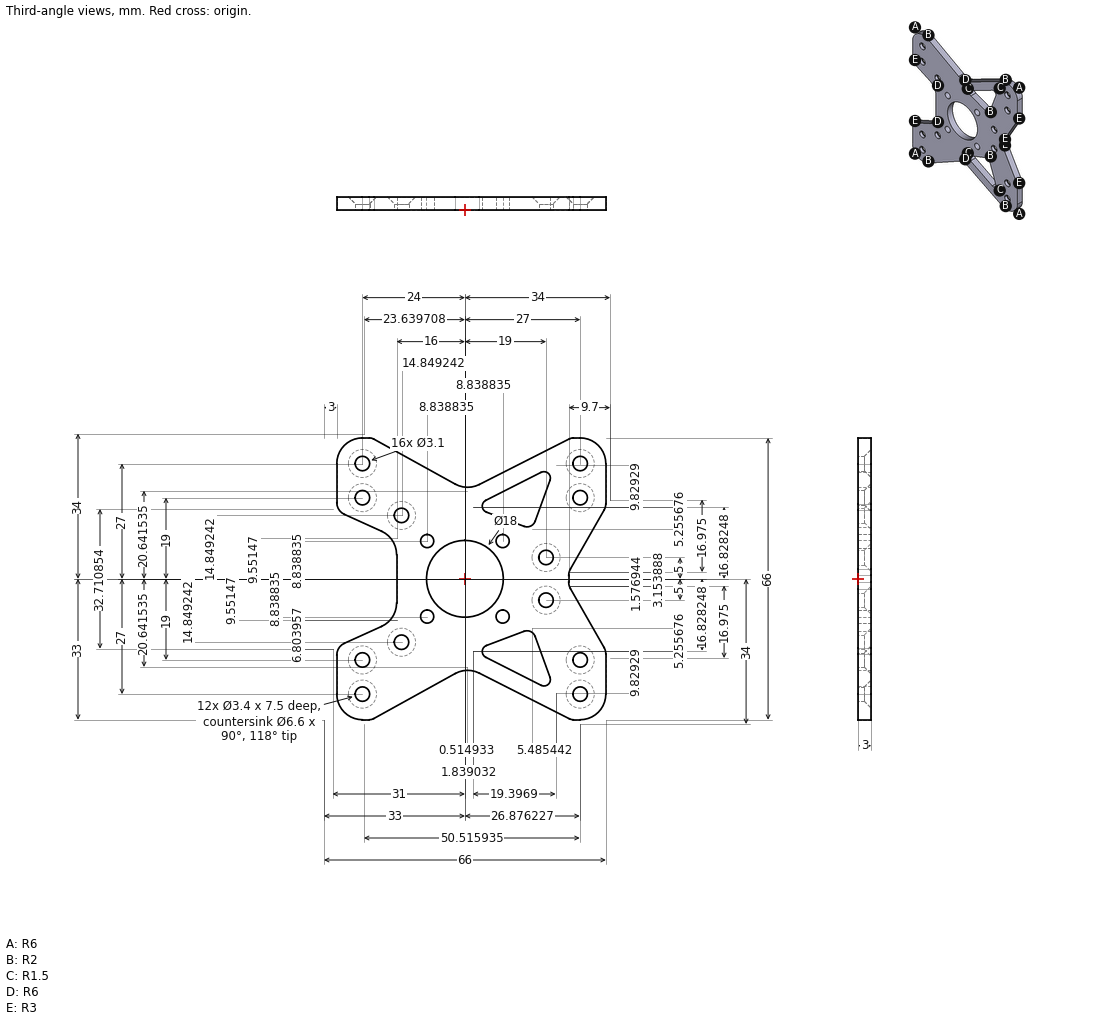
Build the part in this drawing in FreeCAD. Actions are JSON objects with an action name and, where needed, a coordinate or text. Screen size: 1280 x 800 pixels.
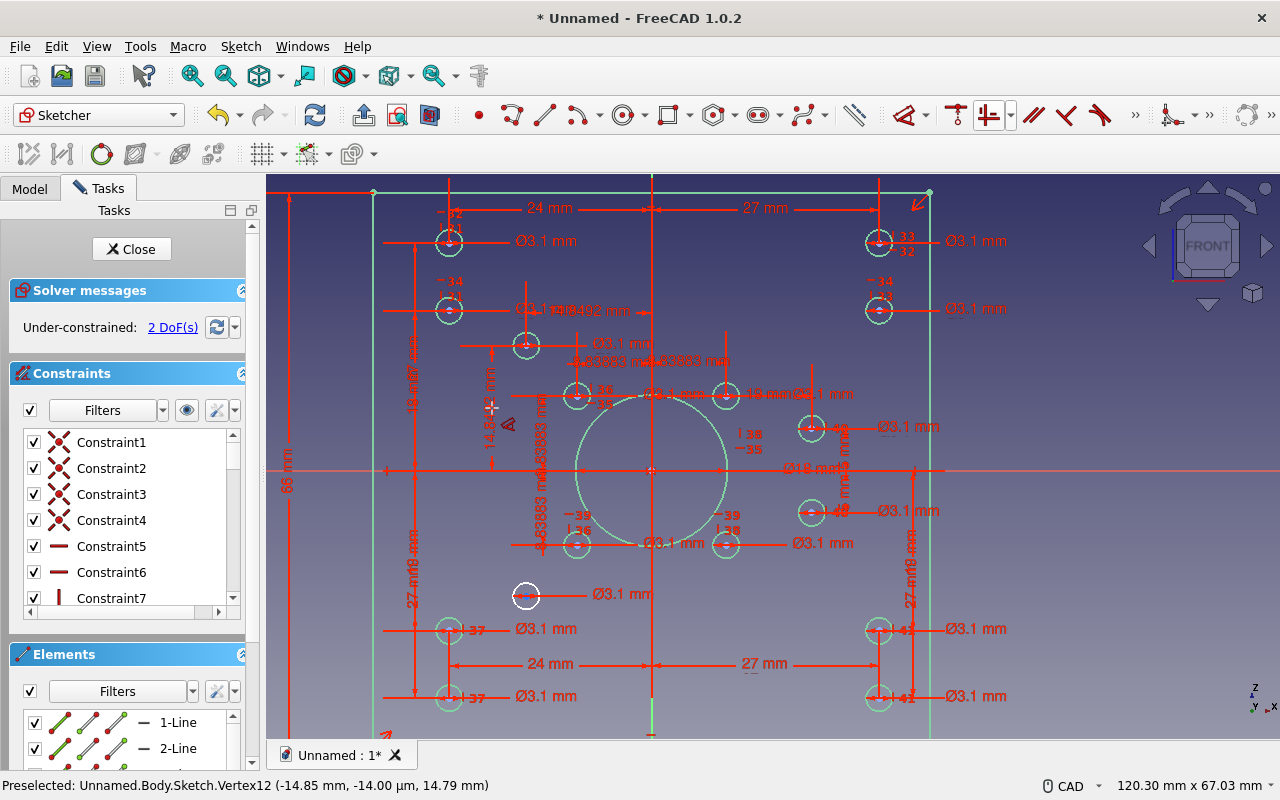
{"action": "left_click", "coordinate": [526, 596]}
{"action": "left_click", "coordinate": [589, 630]}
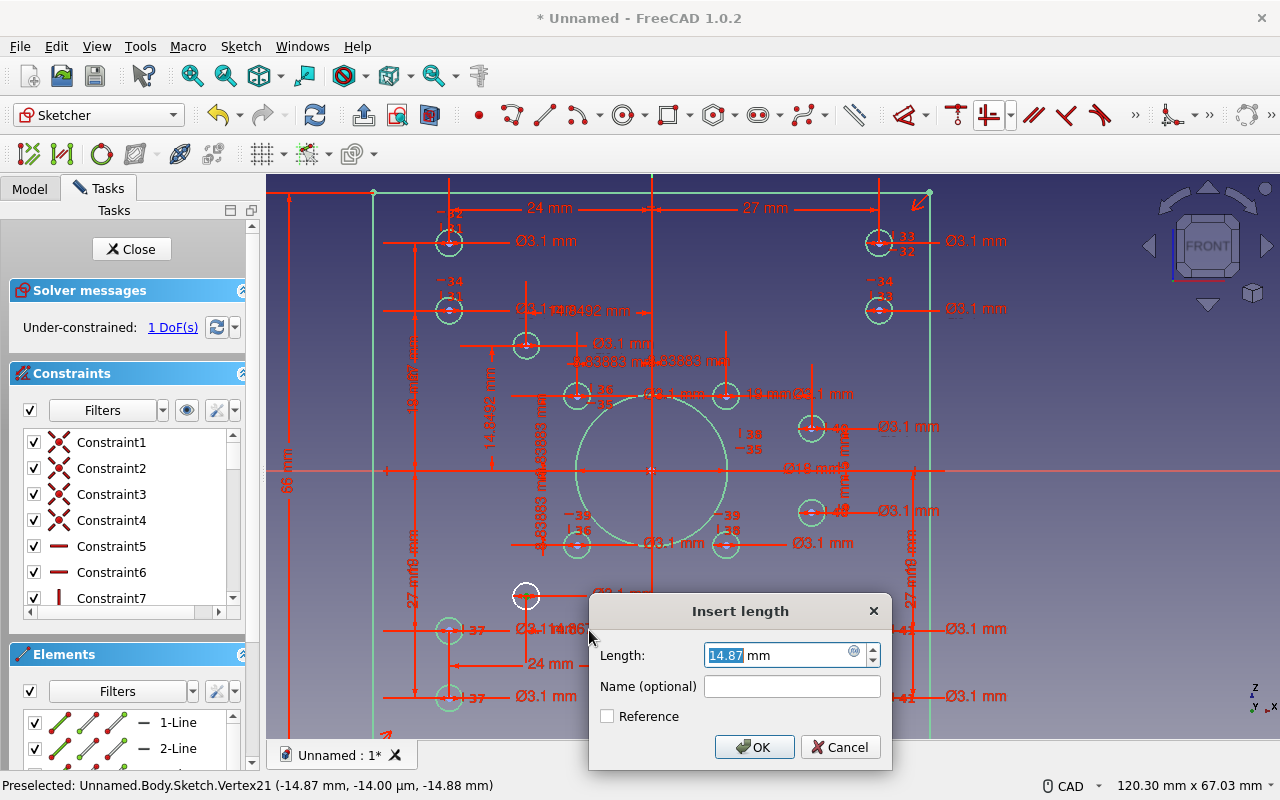
{"action": "type", "text": "14.849242"}
{"action": "key", "text": "Return"}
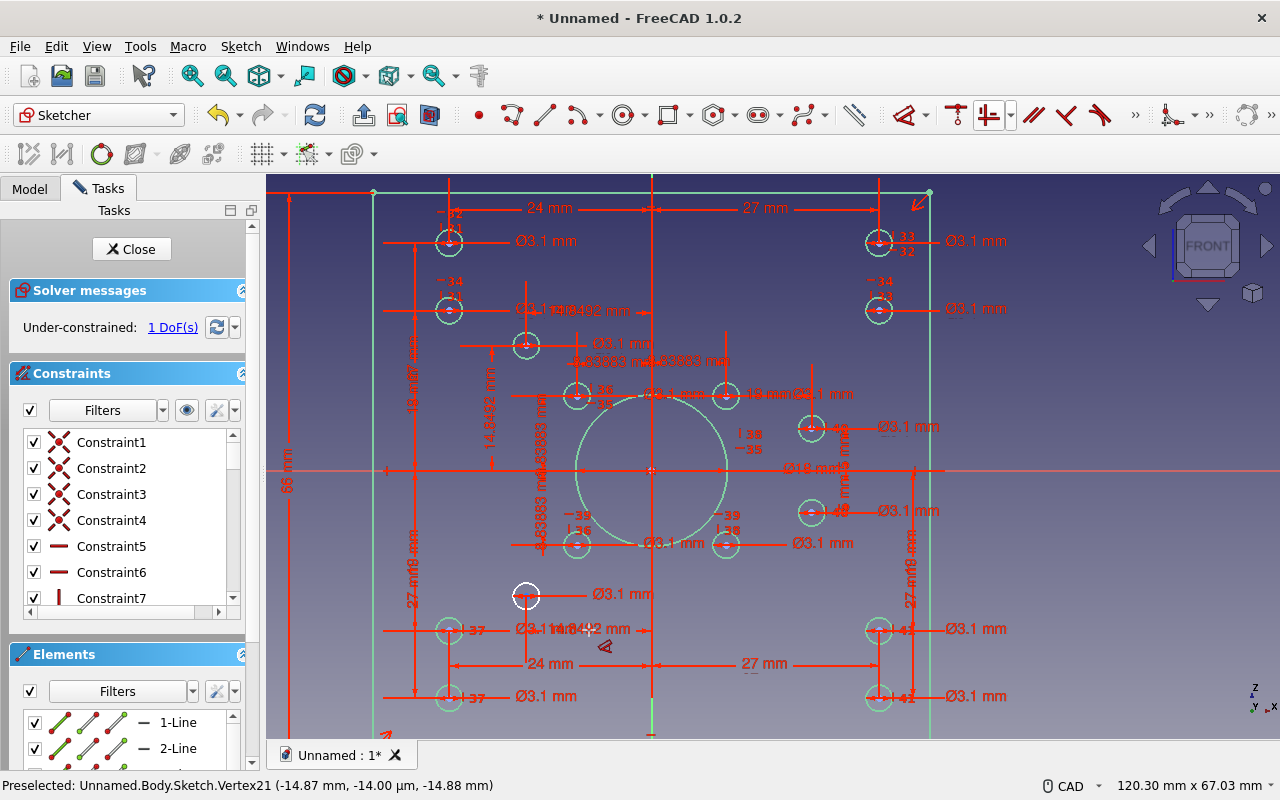
{"action": "left_click", "coordinate": [526, 596]}
{"action": "left_click", "coordinate": [492, 533]}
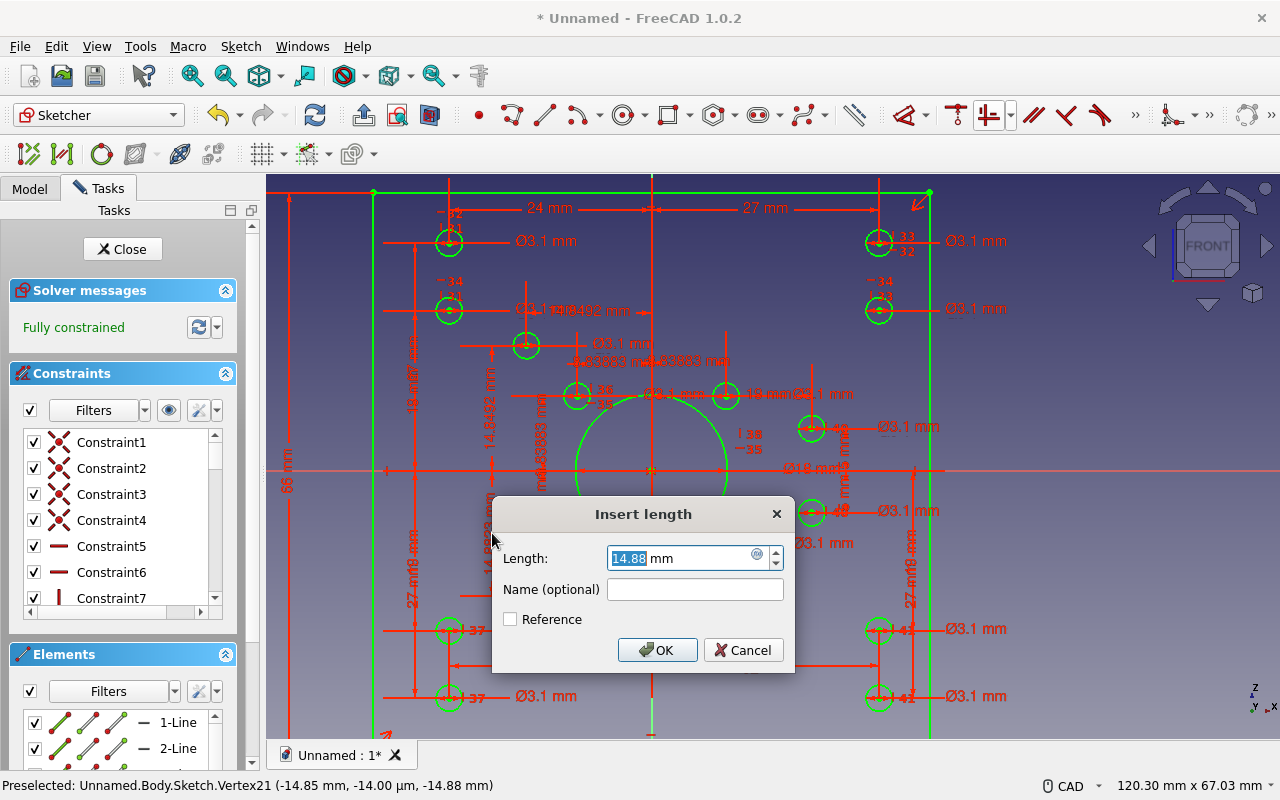
{"action": "type", "text": "14.849242"}
{"action": "key", "text": "Return"}
{"action": "key", "text": "Escape"}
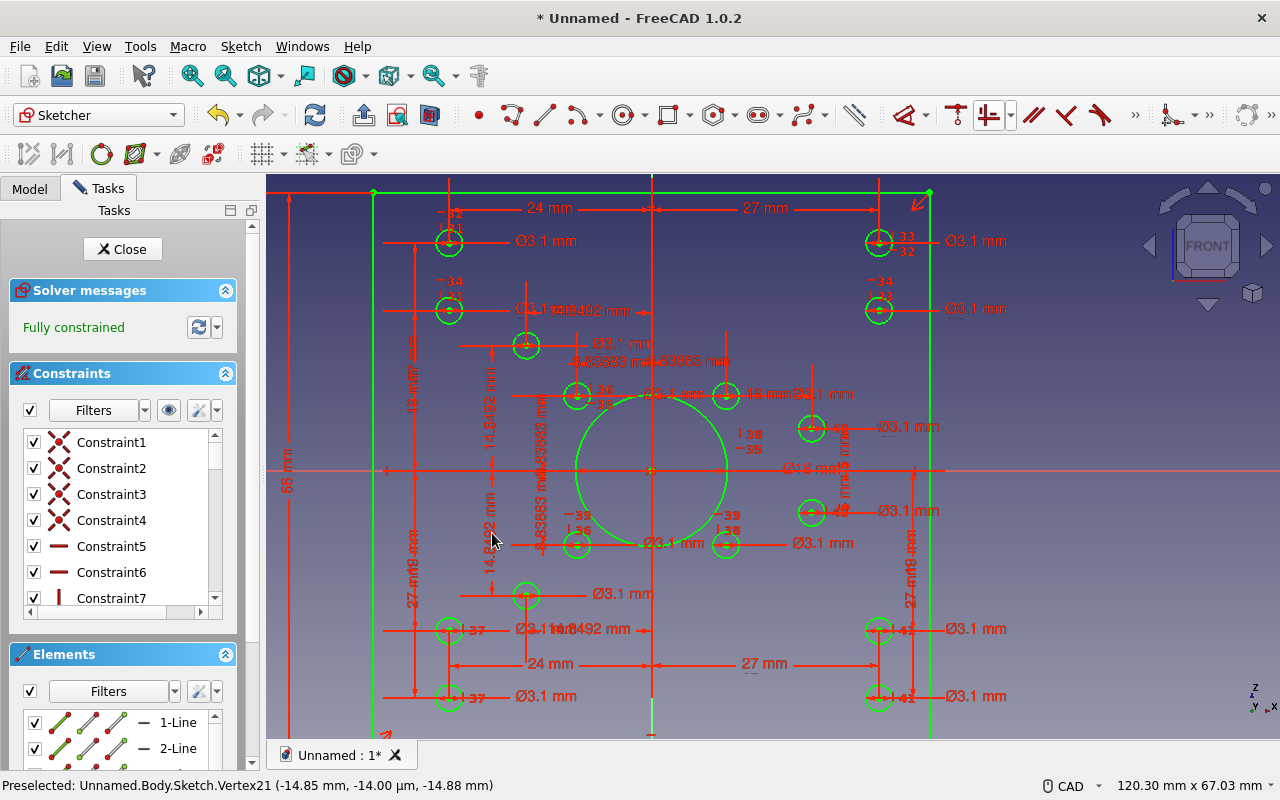
{"action": "left_click", "coordinate": [123, 249]}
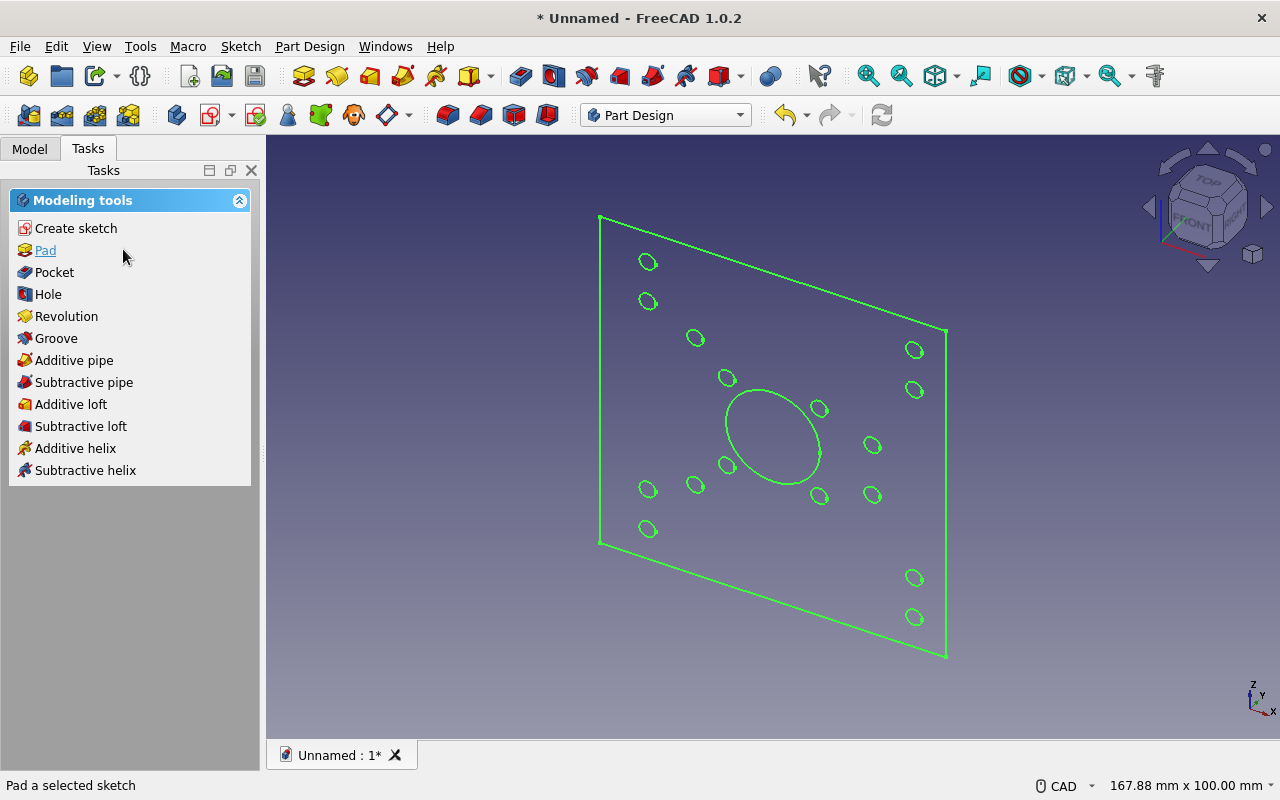
{"action": "left_click", "coordinate": [304, 76]}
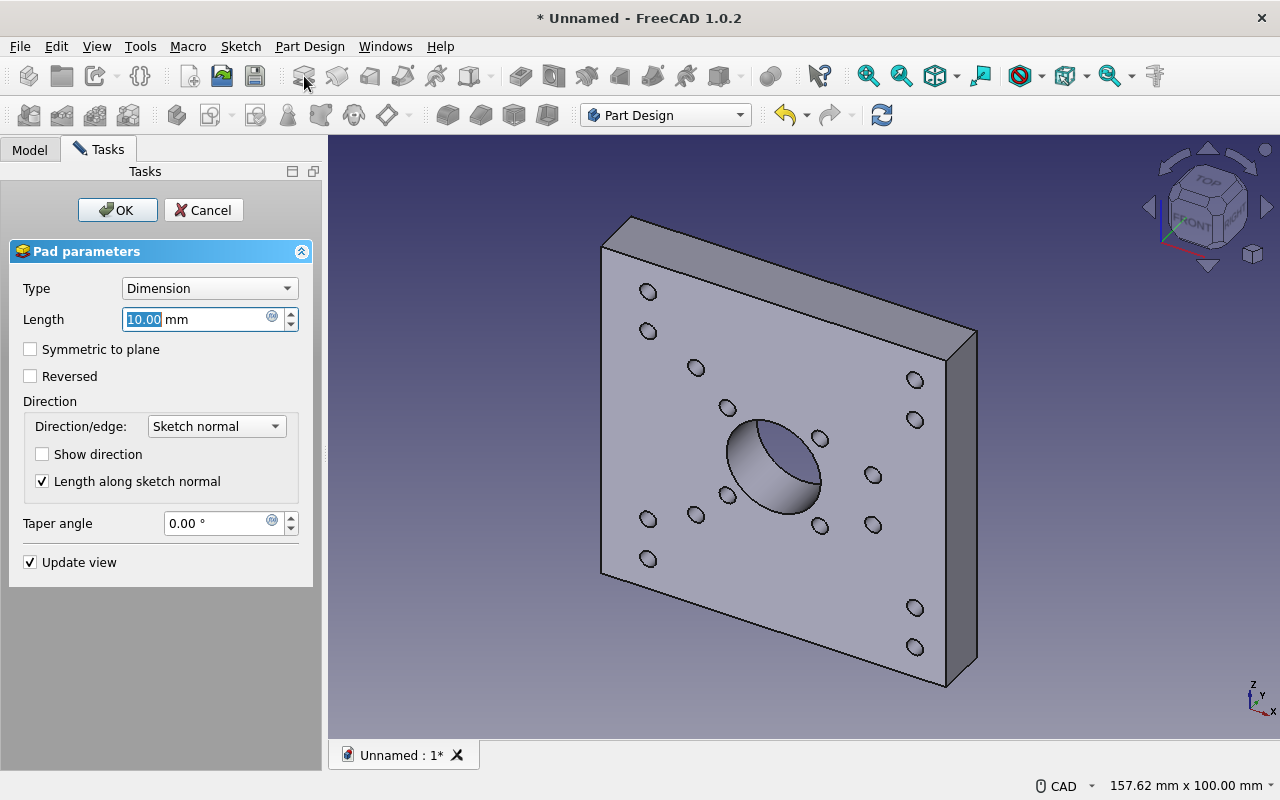
{"action": "type", "text": "3"}
{"action": "key", "text": "Tab"}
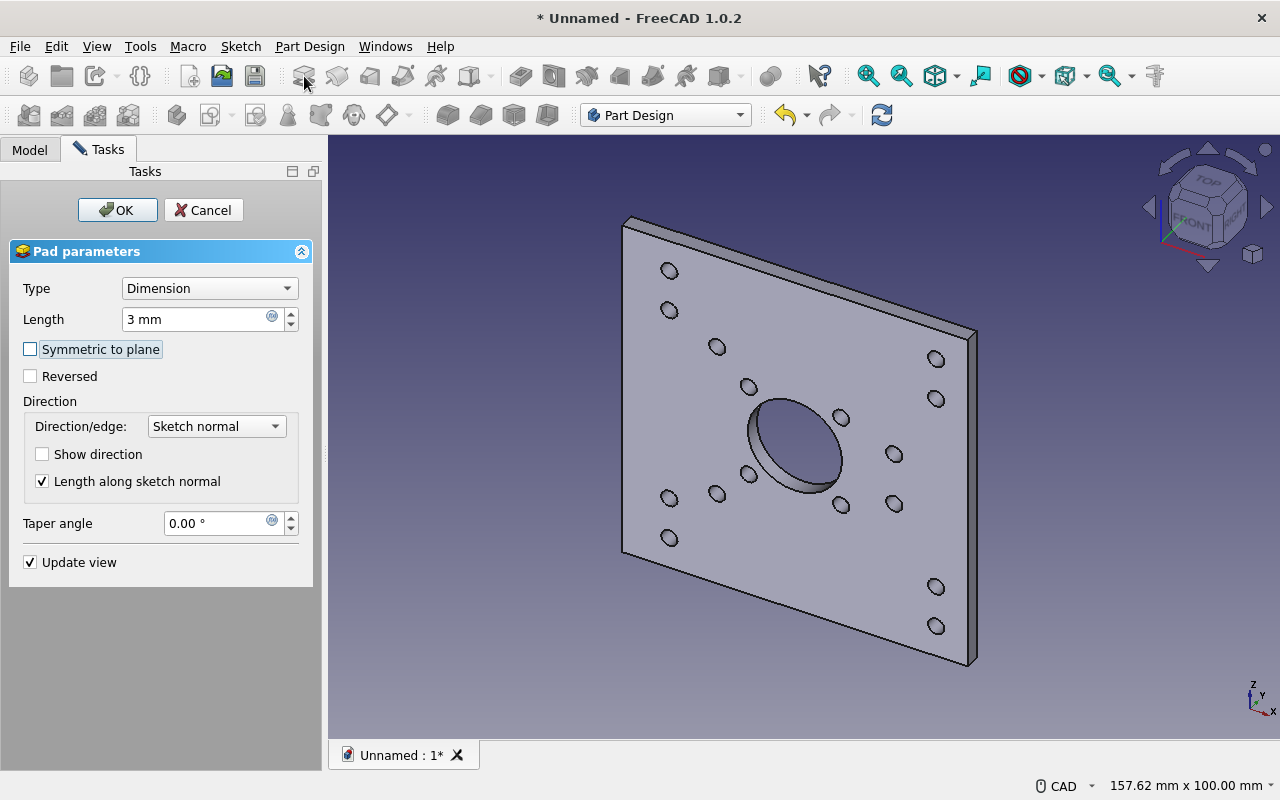
{"action": "left_click", "coordinate": [31, 376]}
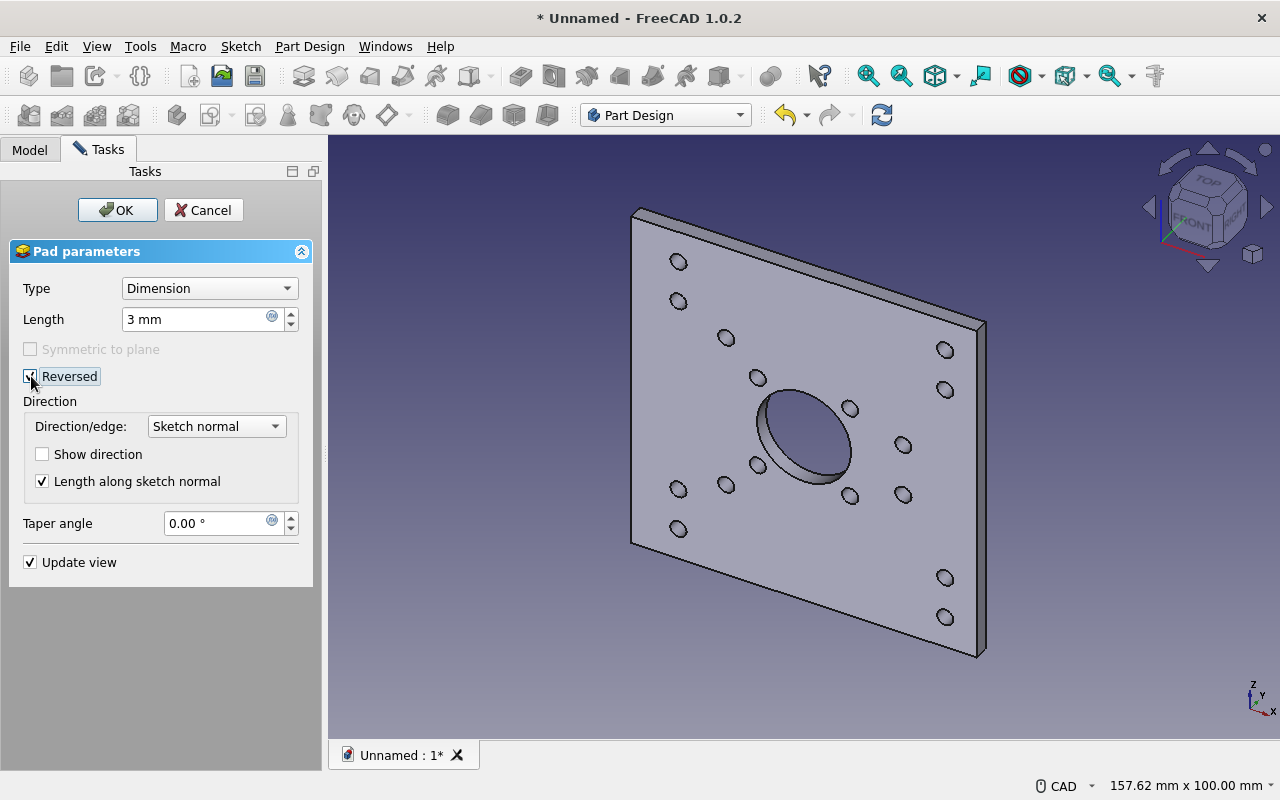
{"action": "left_click", "coordinate": [118, 210]}